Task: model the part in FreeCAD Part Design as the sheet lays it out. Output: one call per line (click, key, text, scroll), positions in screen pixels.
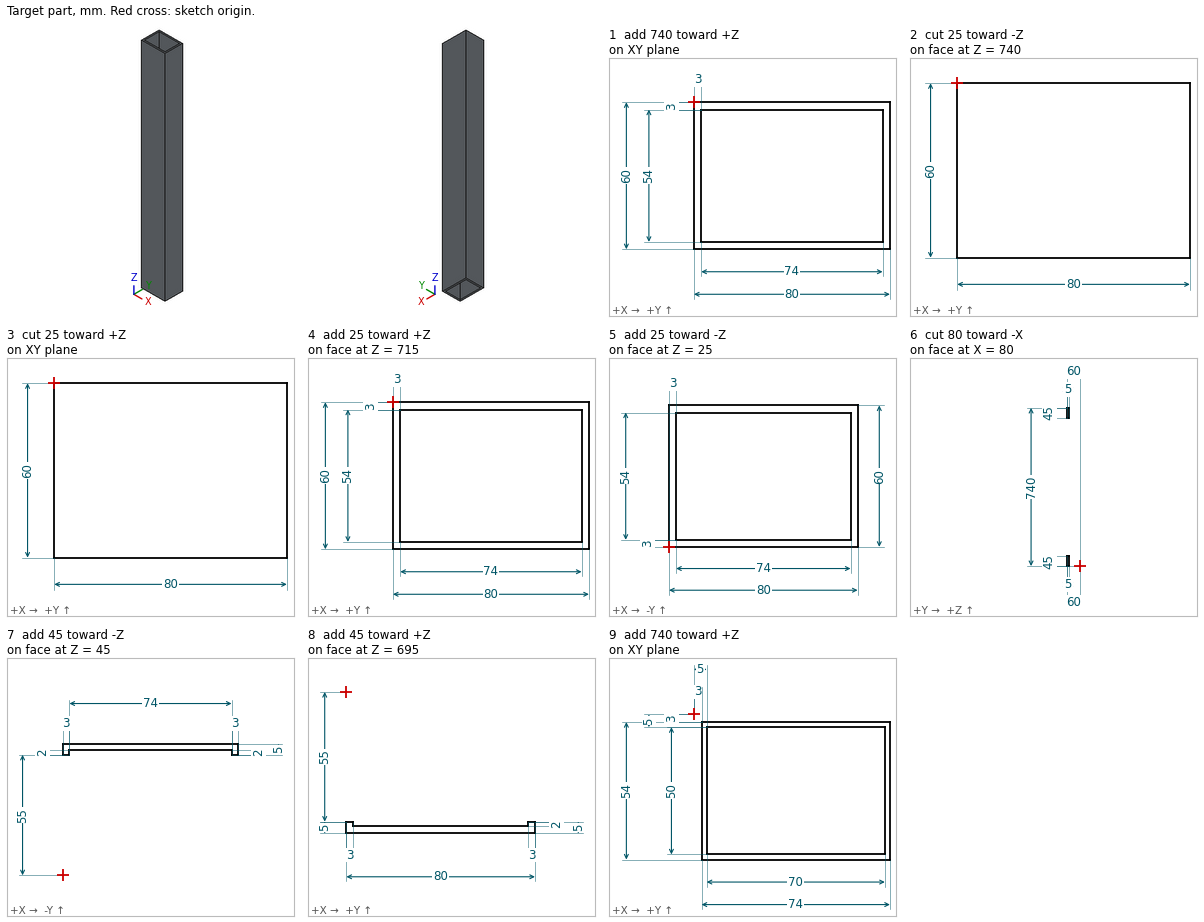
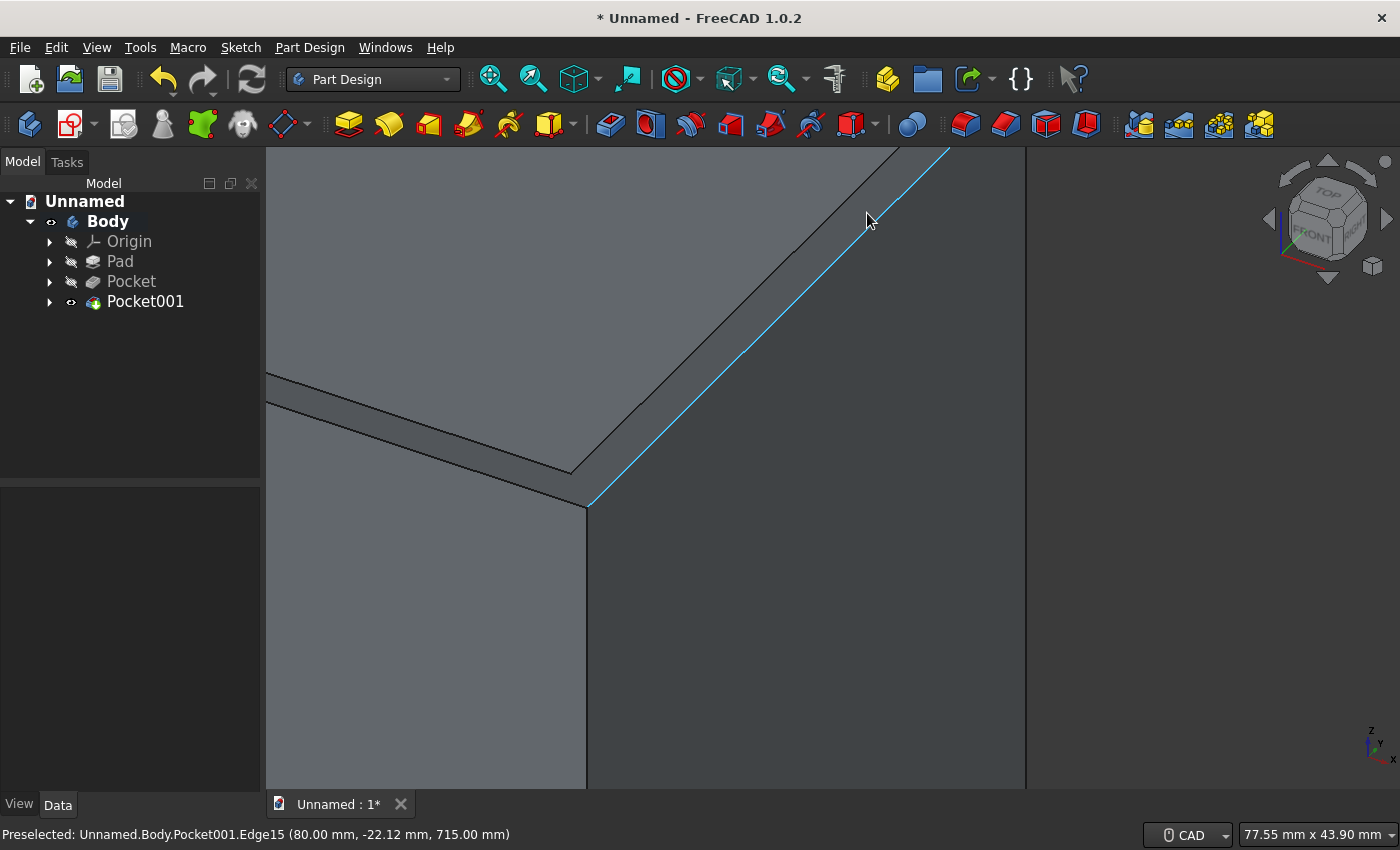
click(859, 220)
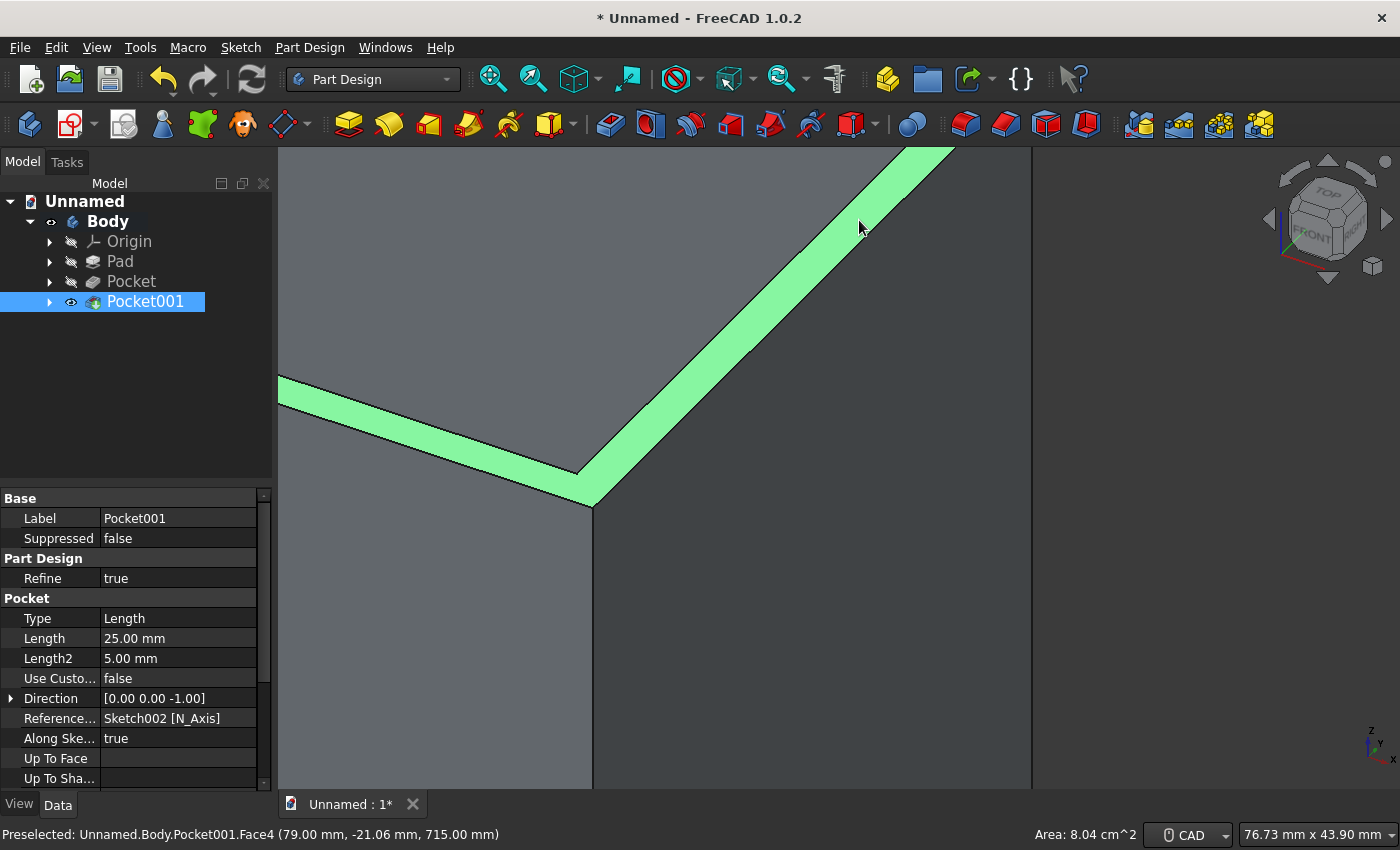
click(70, 124)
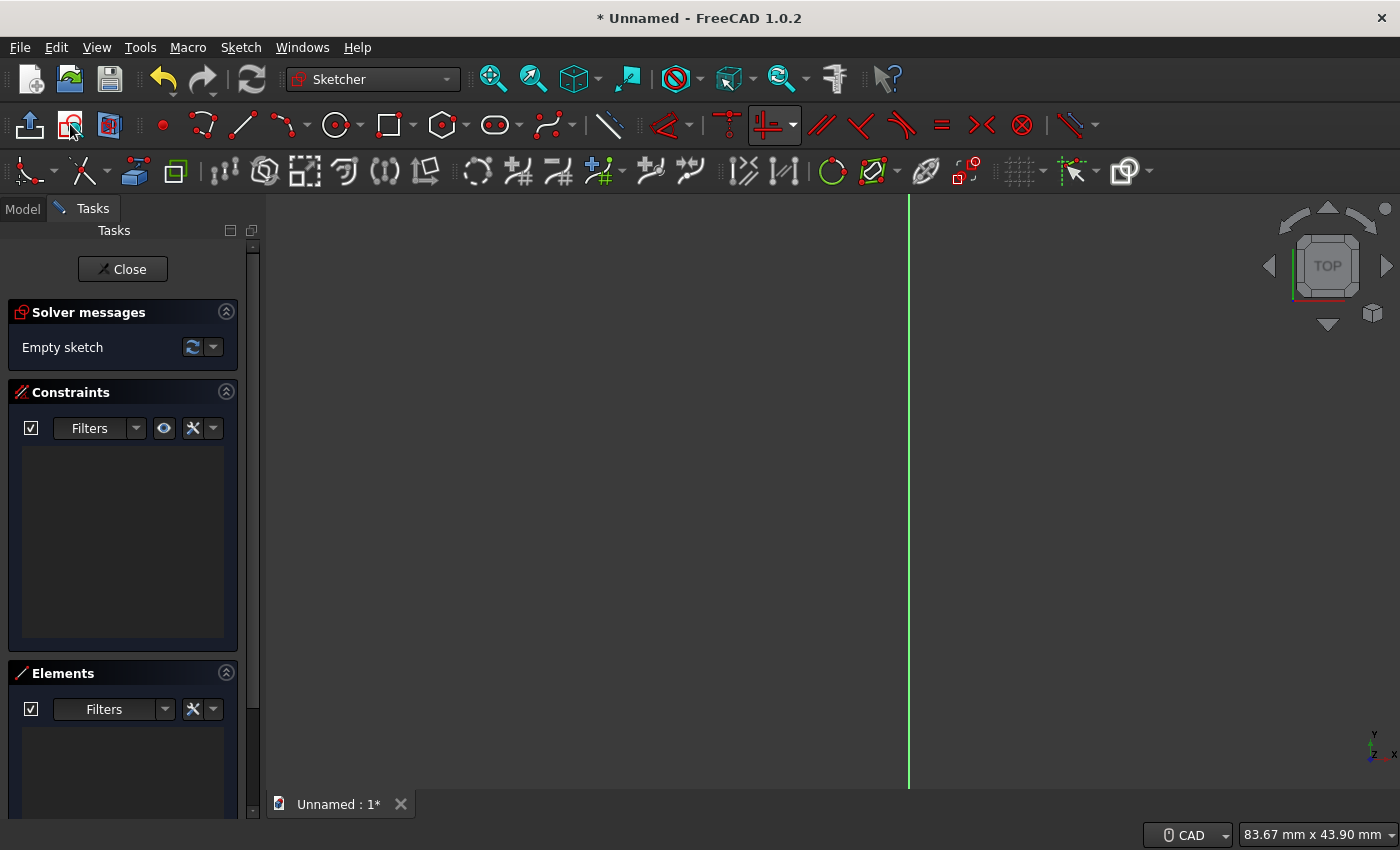
scroll(764, 492, down, 5)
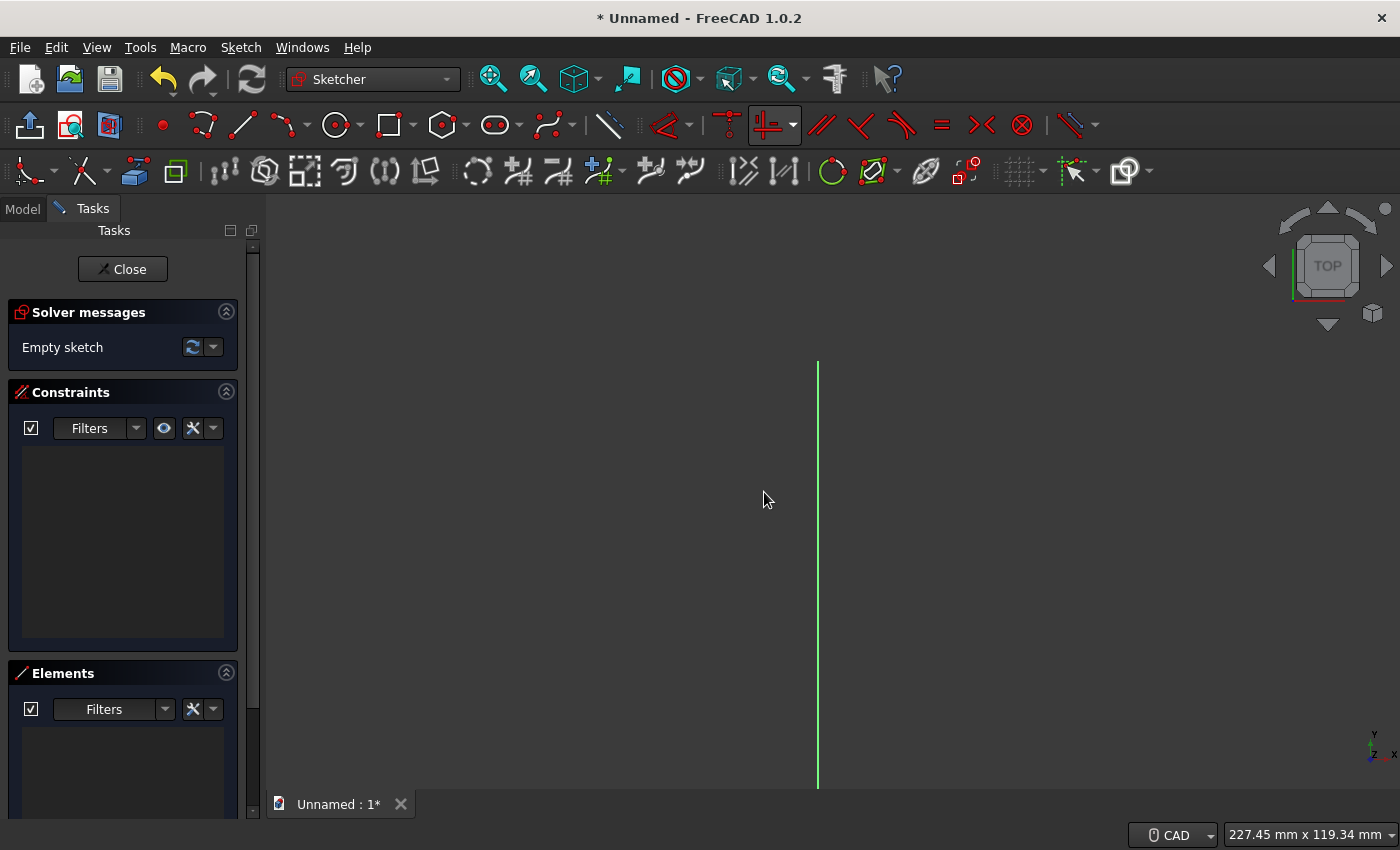
scroll(764, 492, down, 5)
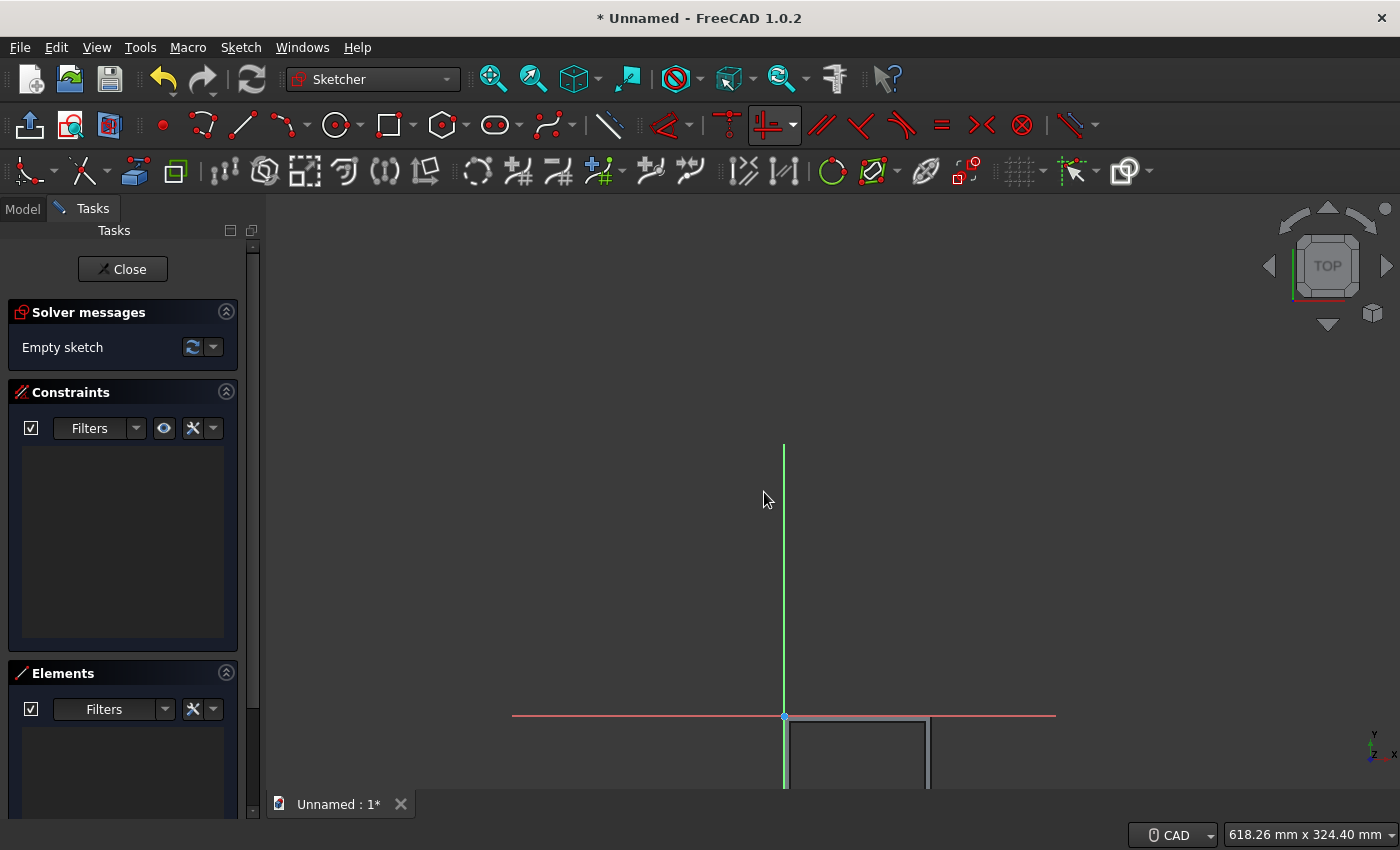
scroll(764, 492, down, 5)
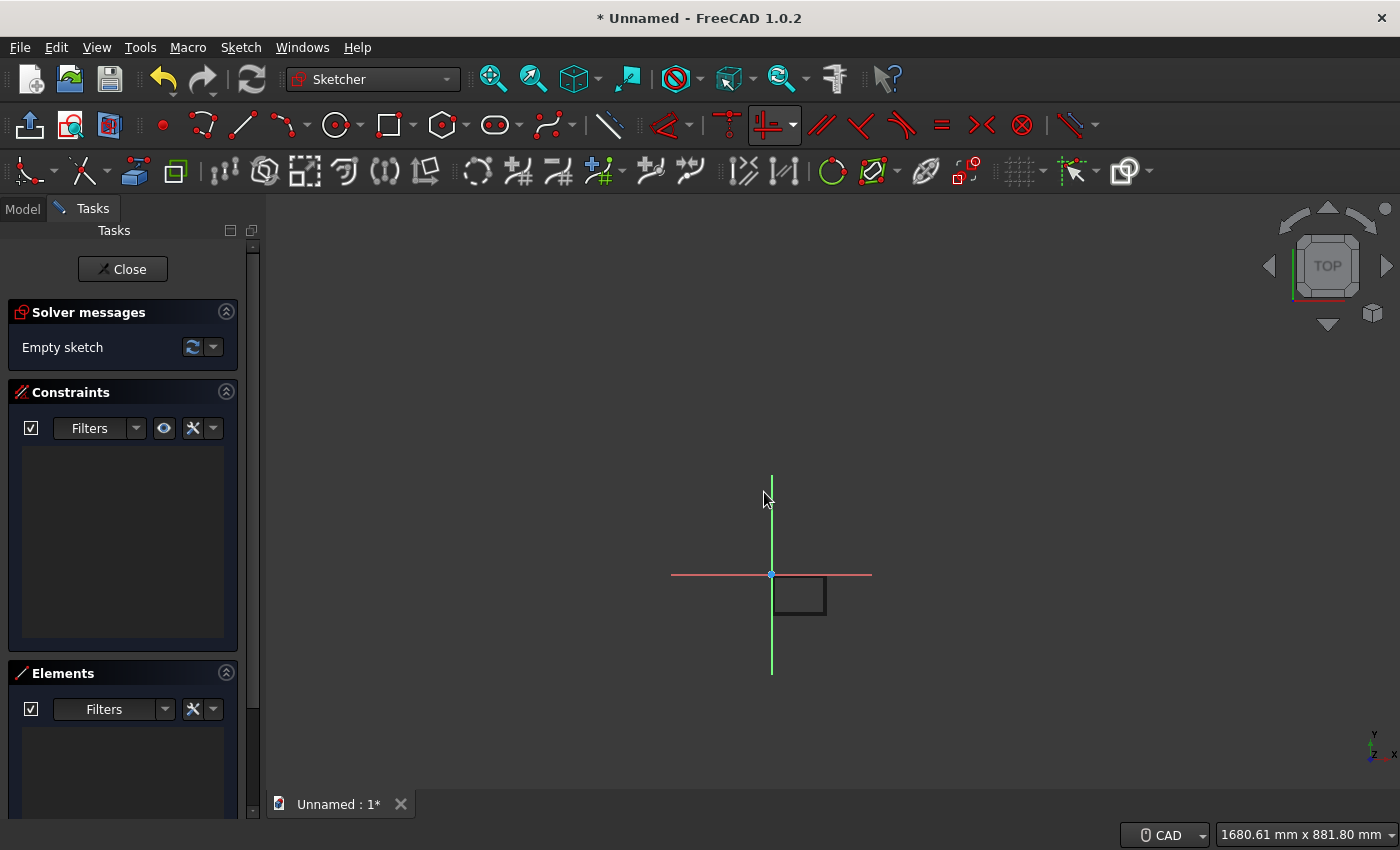
scroll(803, 608, up, 11)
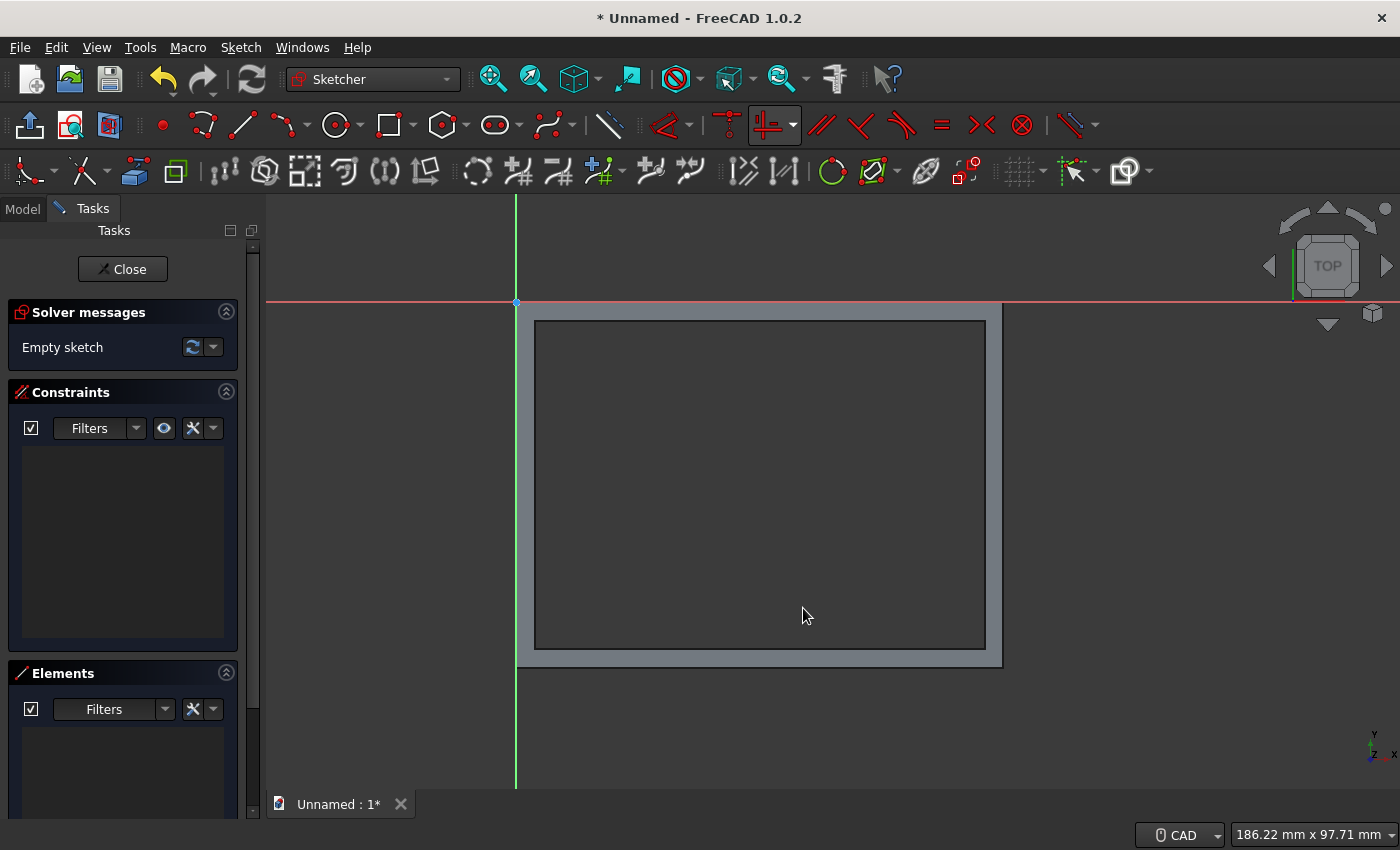
key(g)
key(r)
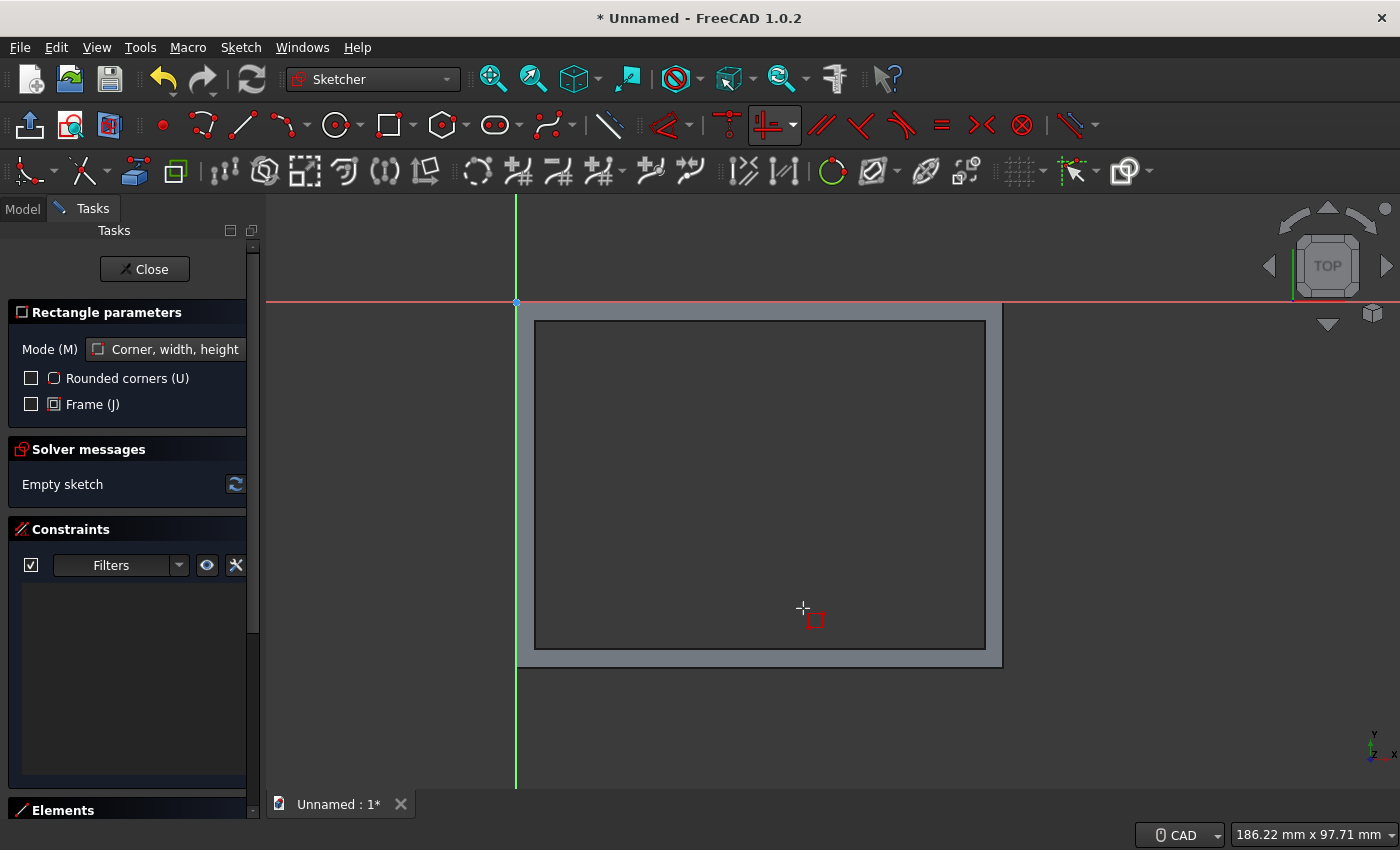
click(516, 302)
click(1003, 668)